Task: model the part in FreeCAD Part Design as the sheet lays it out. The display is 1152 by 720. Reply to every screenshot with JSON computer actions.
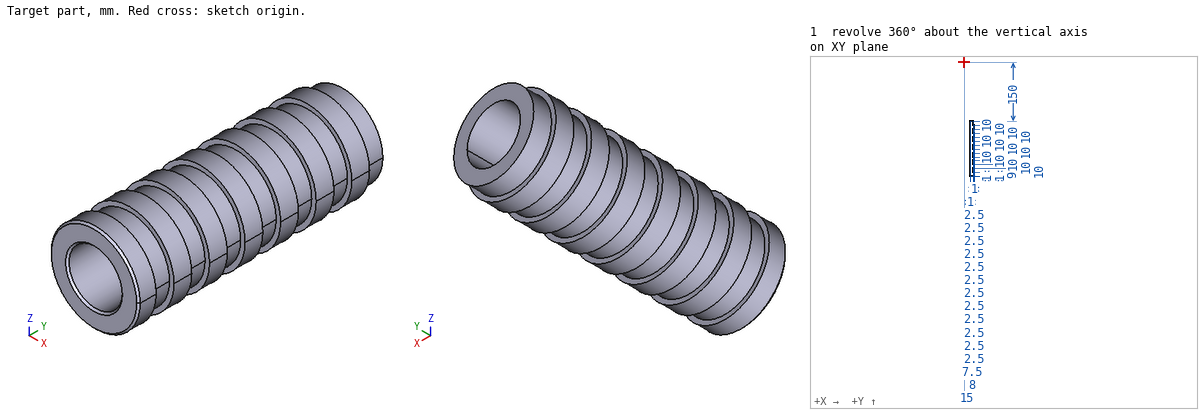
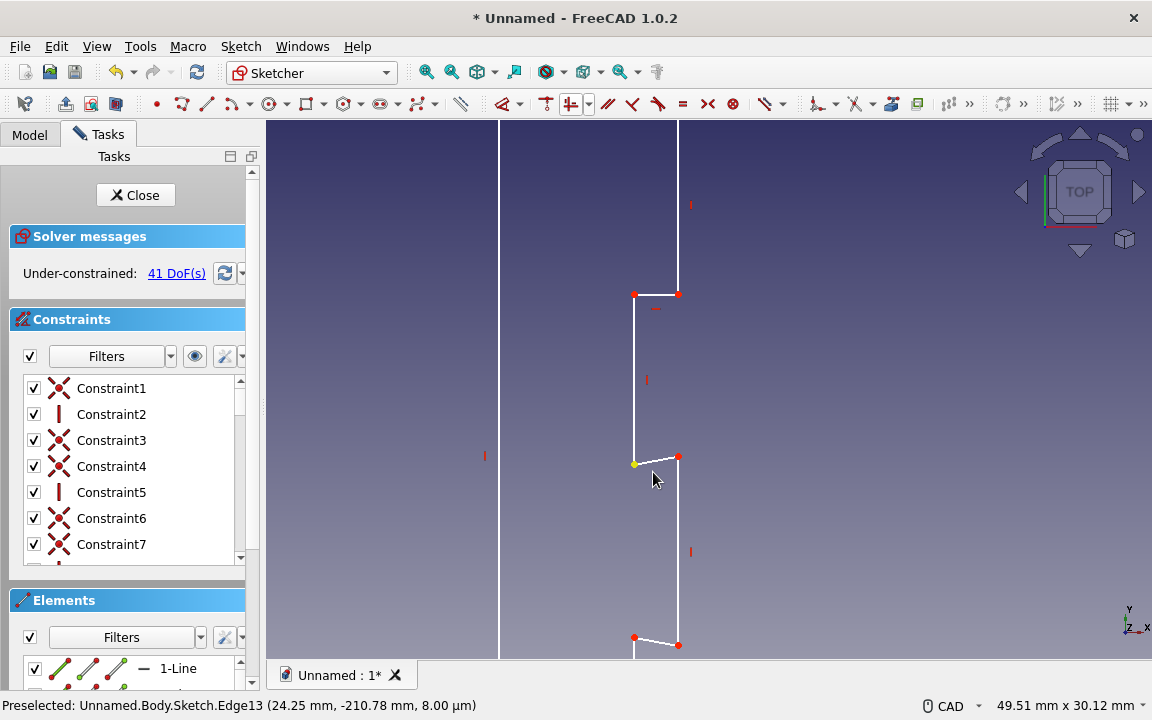
{"action": "left_click", "coordinate": [647, 462]}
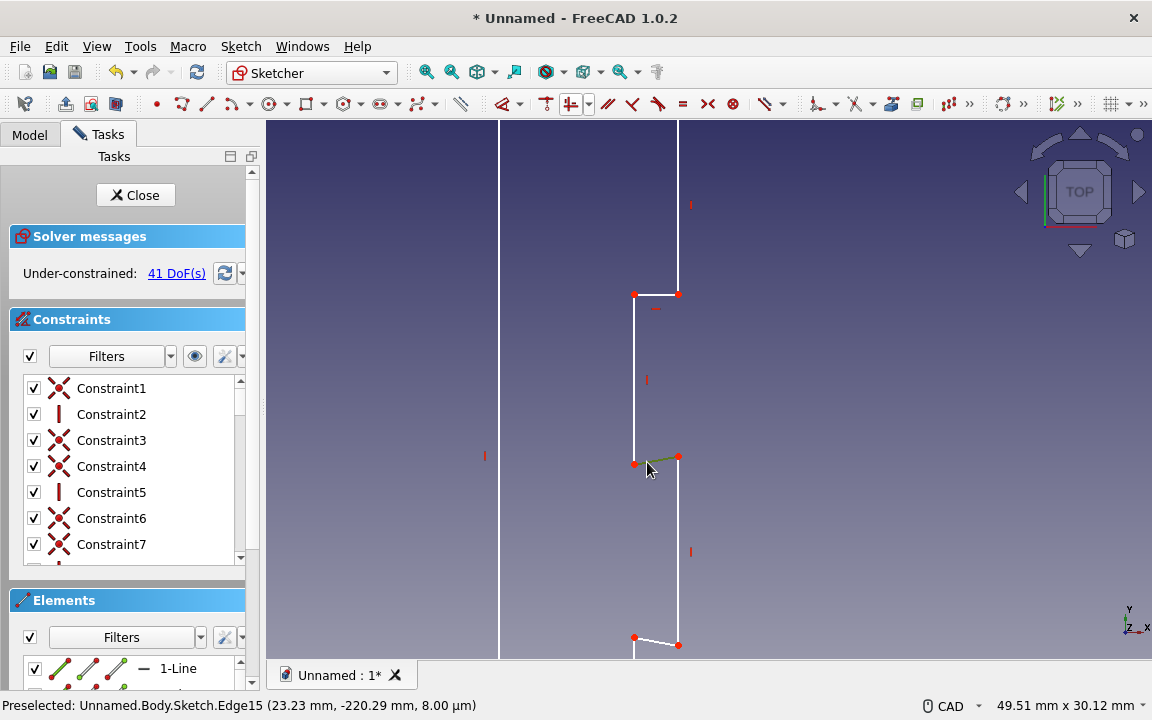
{"action": "key", "text": "h"}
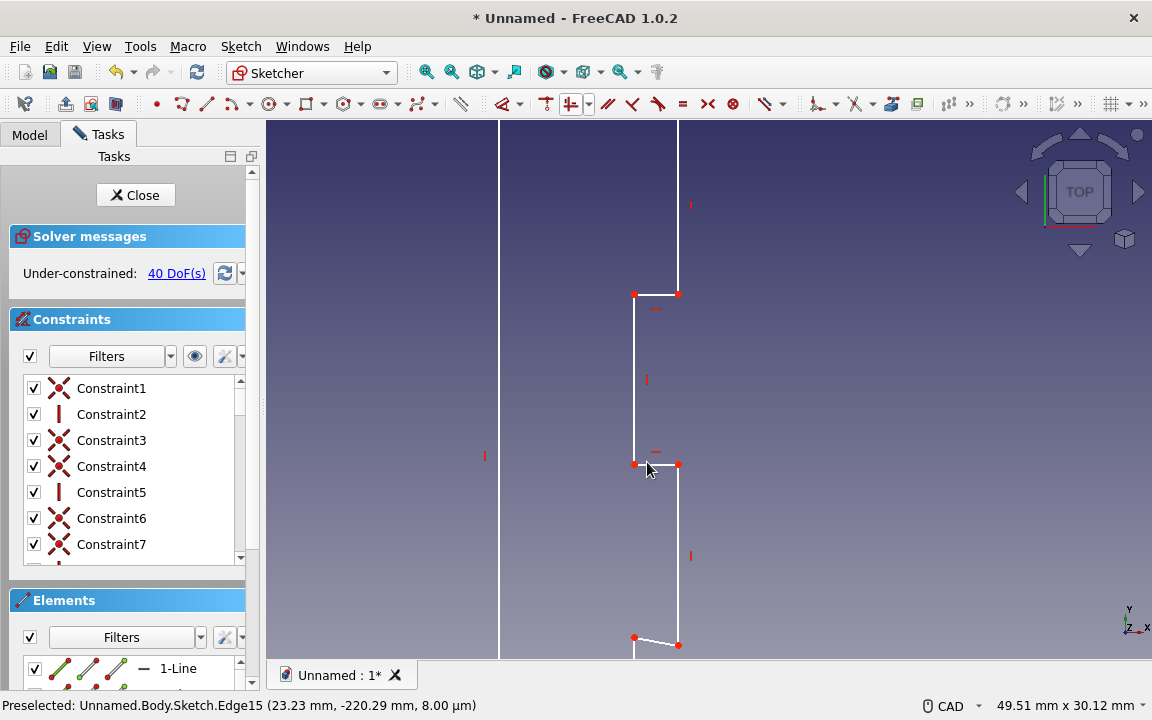
{"action": "scroll", "coordinate": [653, 472], "scroll_direction": "down", "scroll_amount": 14}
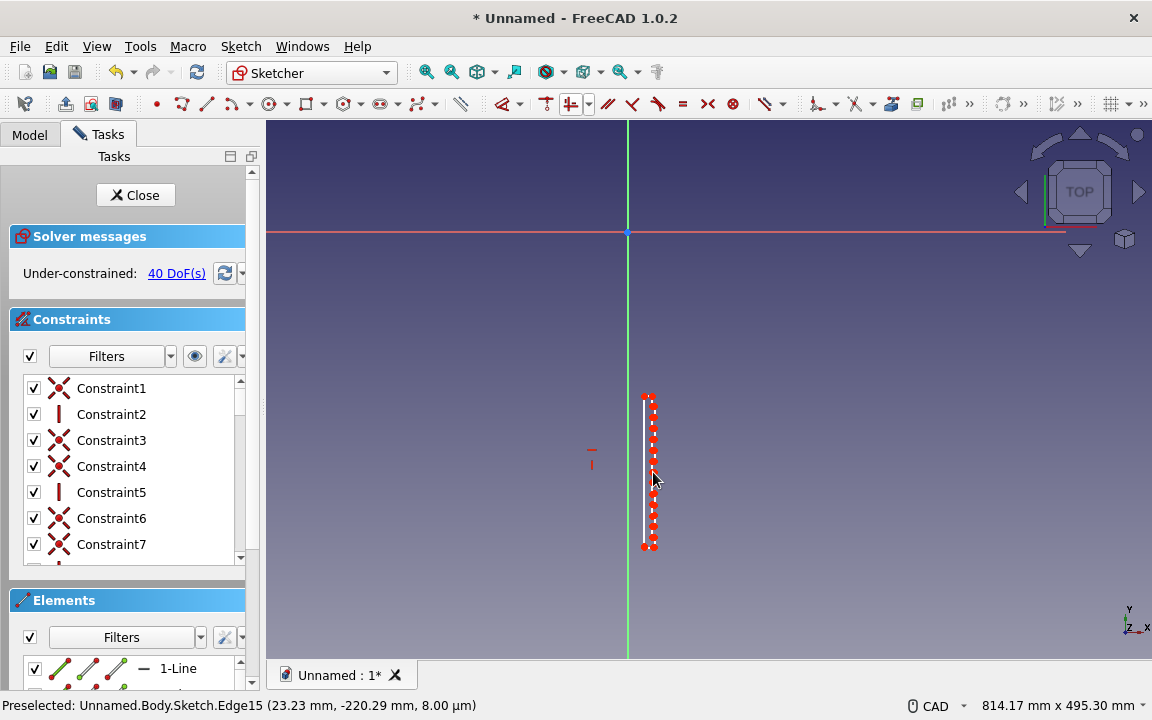
{"action": "scroll", "coordinate": [654, 483], "scroll_direction": "up", "scroll_amount": 14}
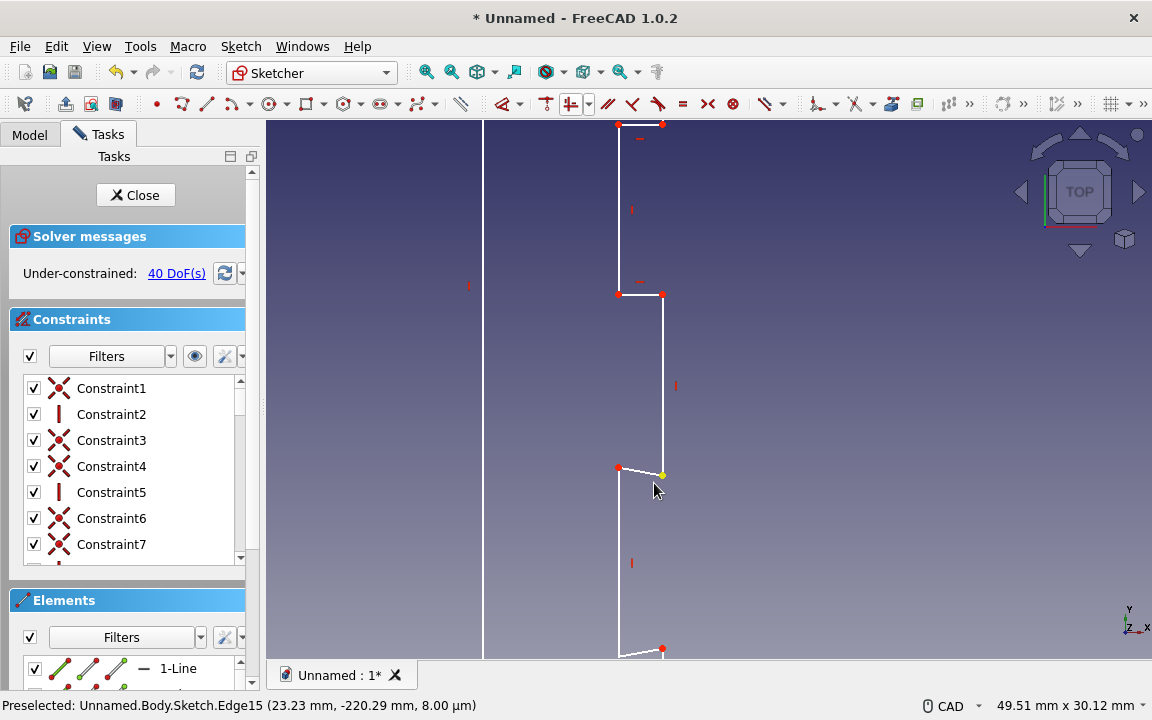
{"action": "left_click", "coordinate": [649, 473]}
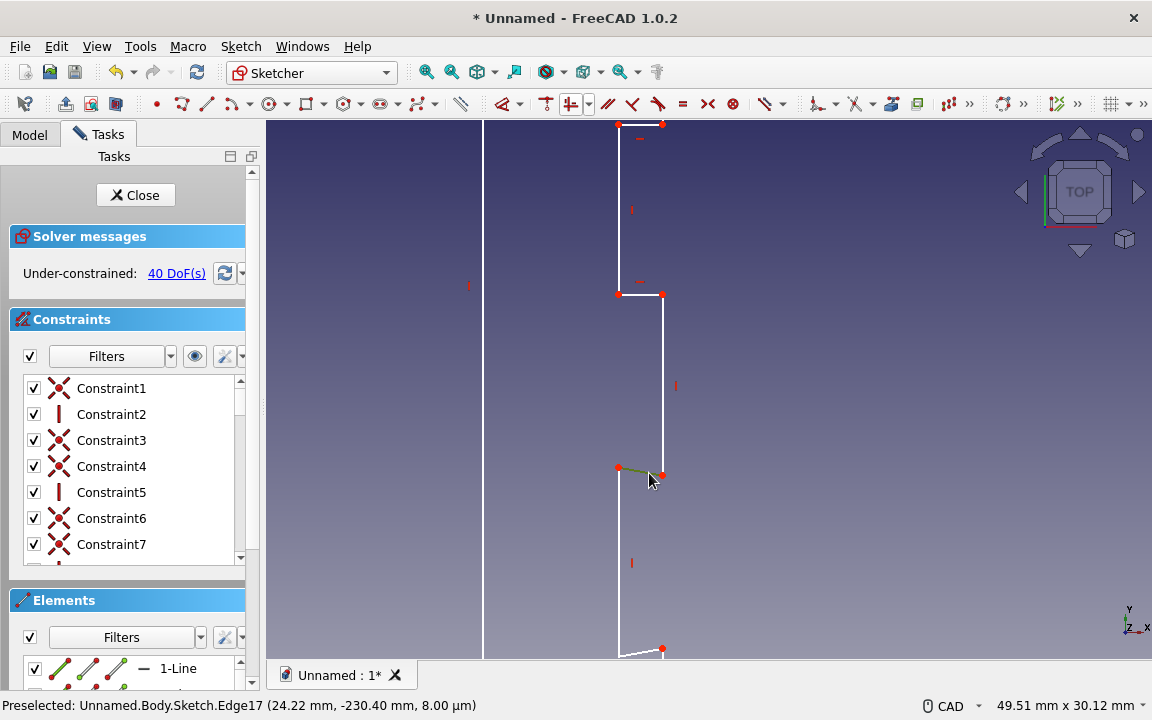
{"action": "key", "text": "h"}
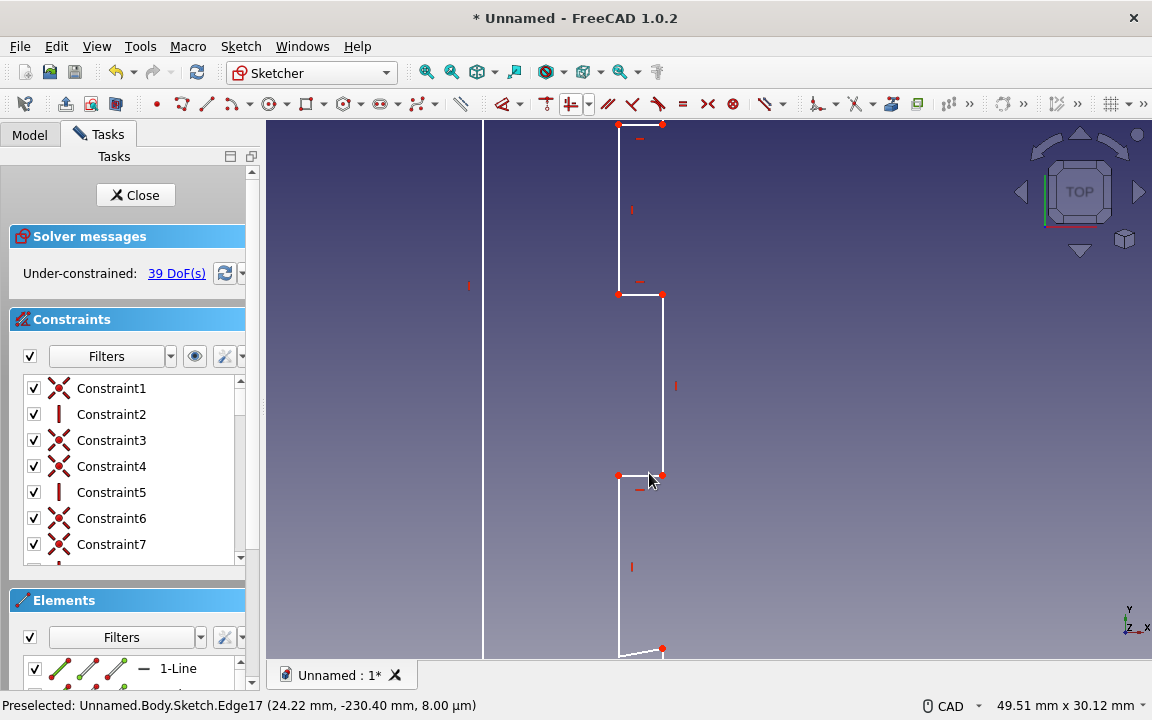
{"action": "scroll", "coordinate": [654, 483], "scroll_direction": "down", "scroll_amount": 14}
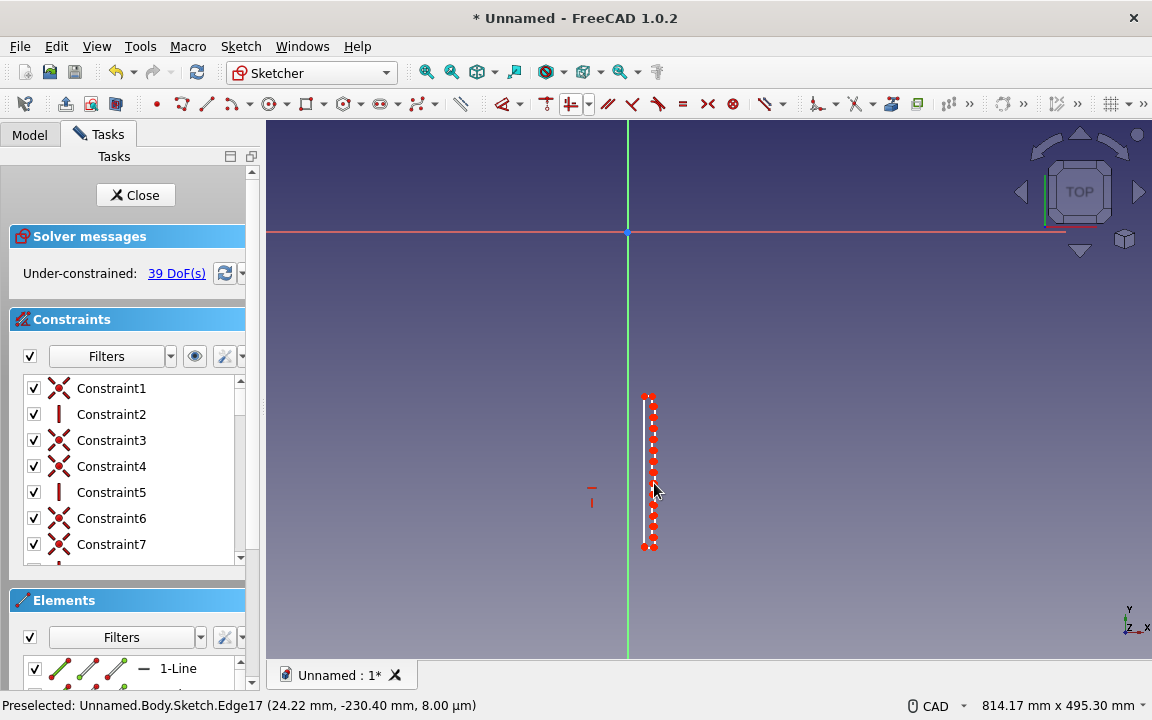
{"action": "scroll", "coordinate": [653, 494], "scroll_direction": "up", "scroll_amount": 14}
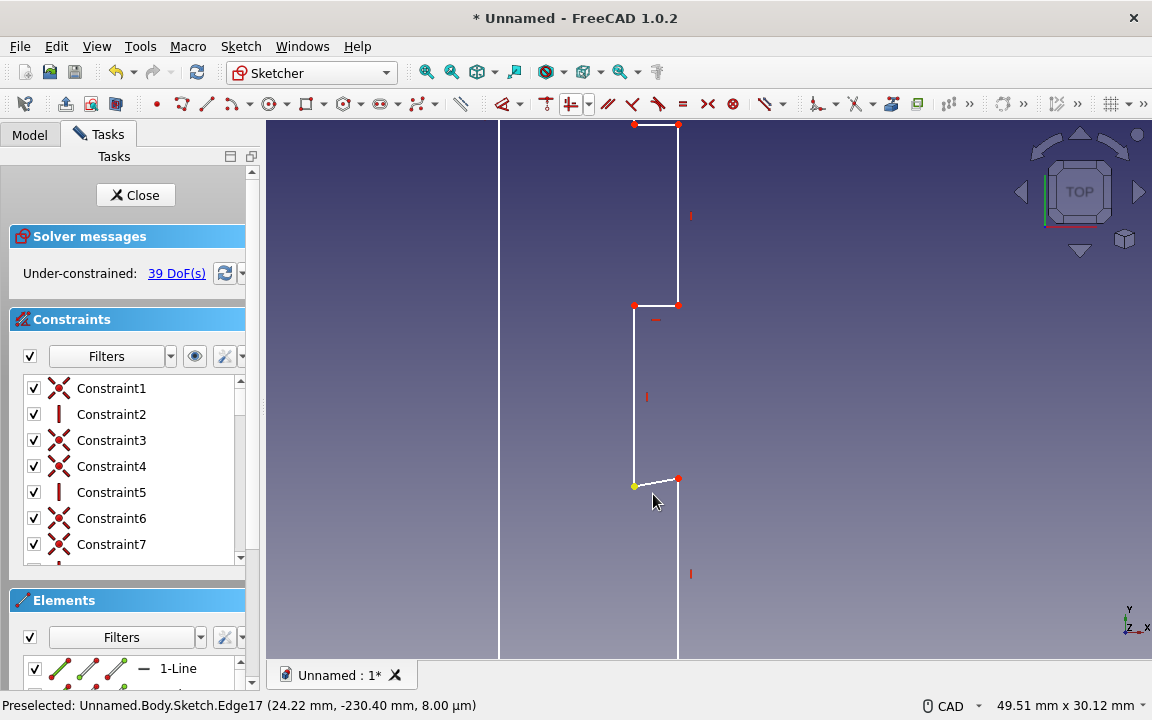
{"action": "left_click", "coordinate": [647, 484]}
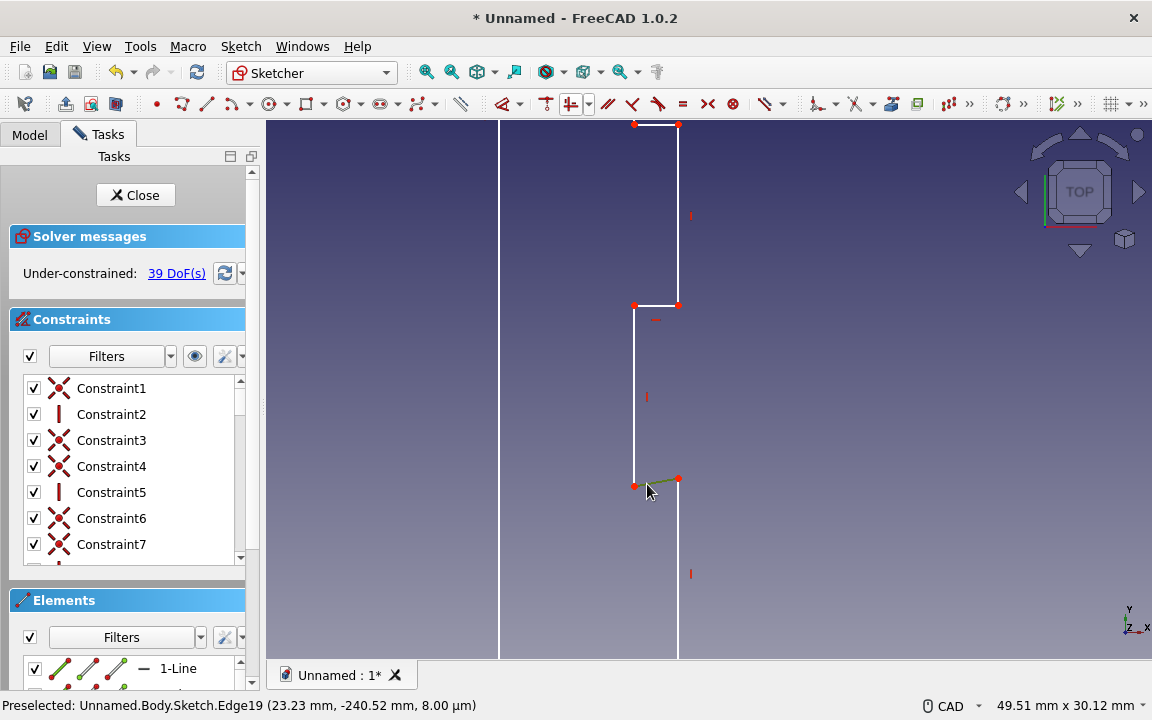
{"action": "key", "text": "h"}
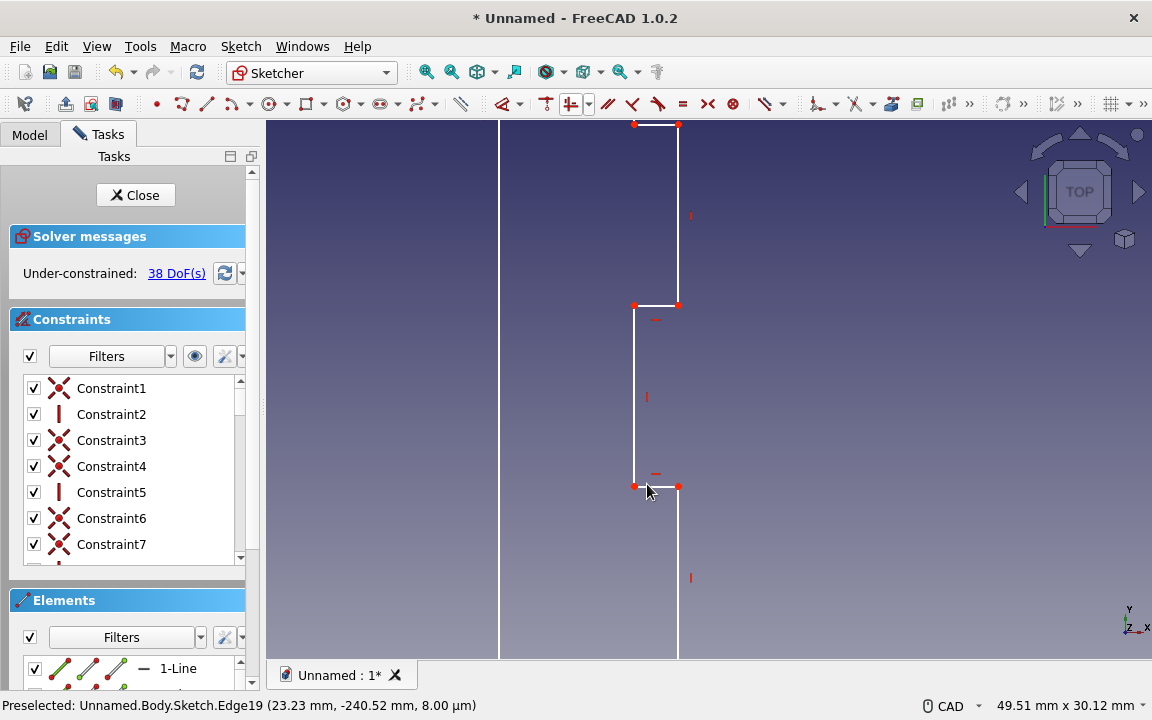
{"action": "scroll", "coordinate": [653, 494], "scroll_direction": "down", "scroll_amount": 14}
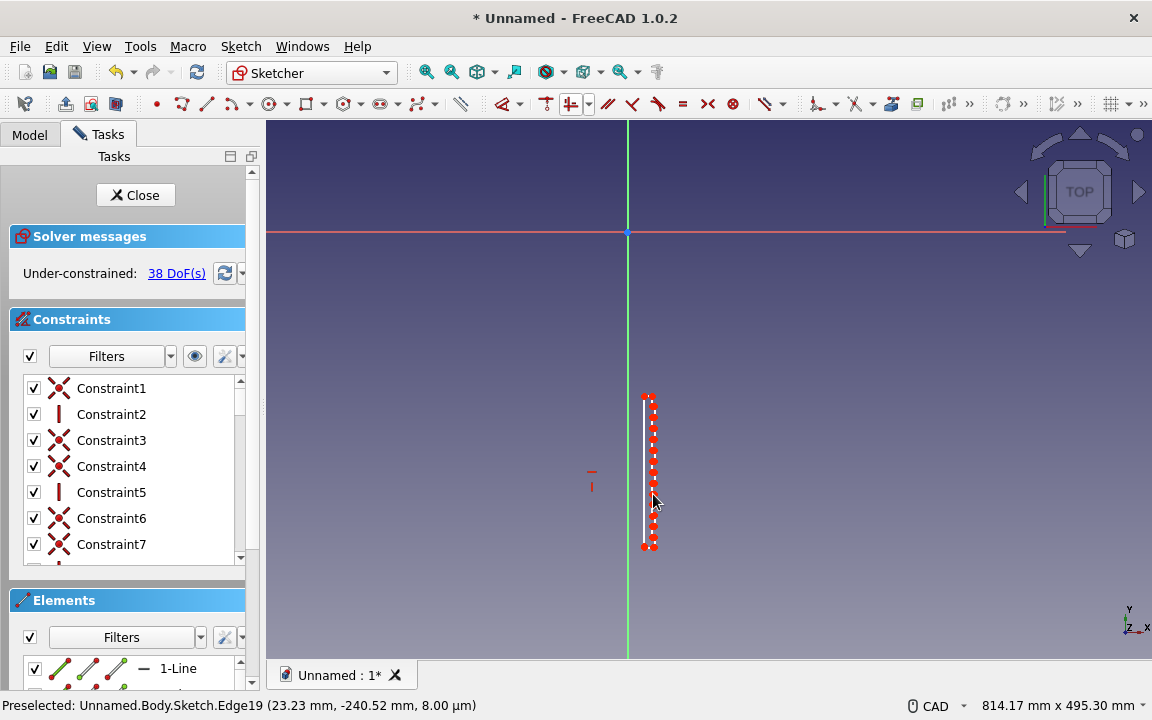
{"action": "scroll", "coordinate": [654, 505], "scroll_direction": "up", "scroll_amount": 14}